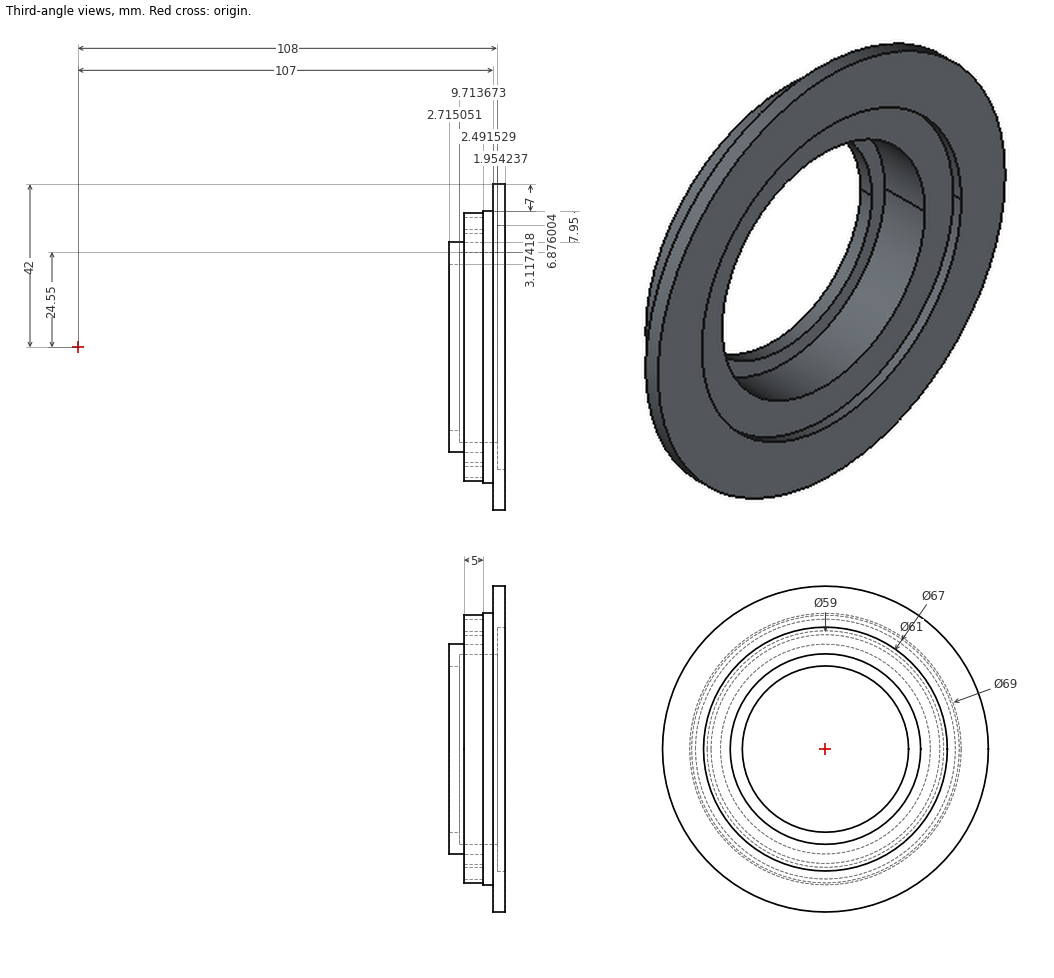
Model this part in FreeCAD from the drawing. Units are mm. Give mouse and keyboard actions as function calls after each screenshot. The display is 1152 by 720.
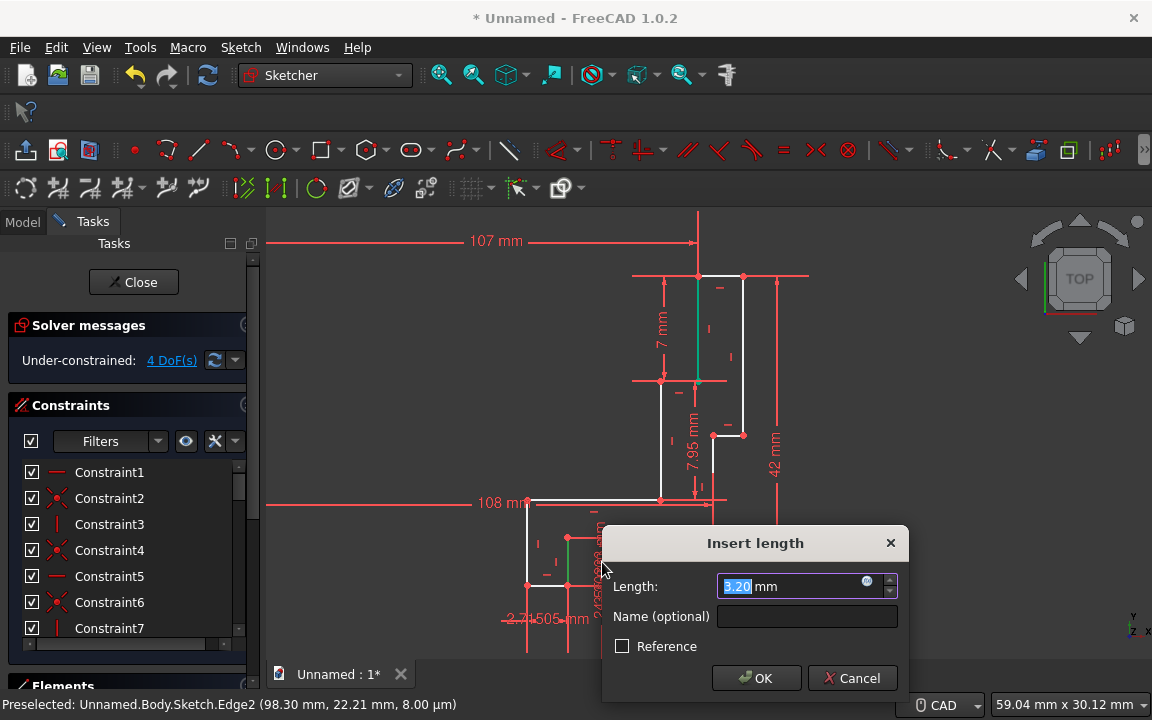
text(3.117418)
key(Return)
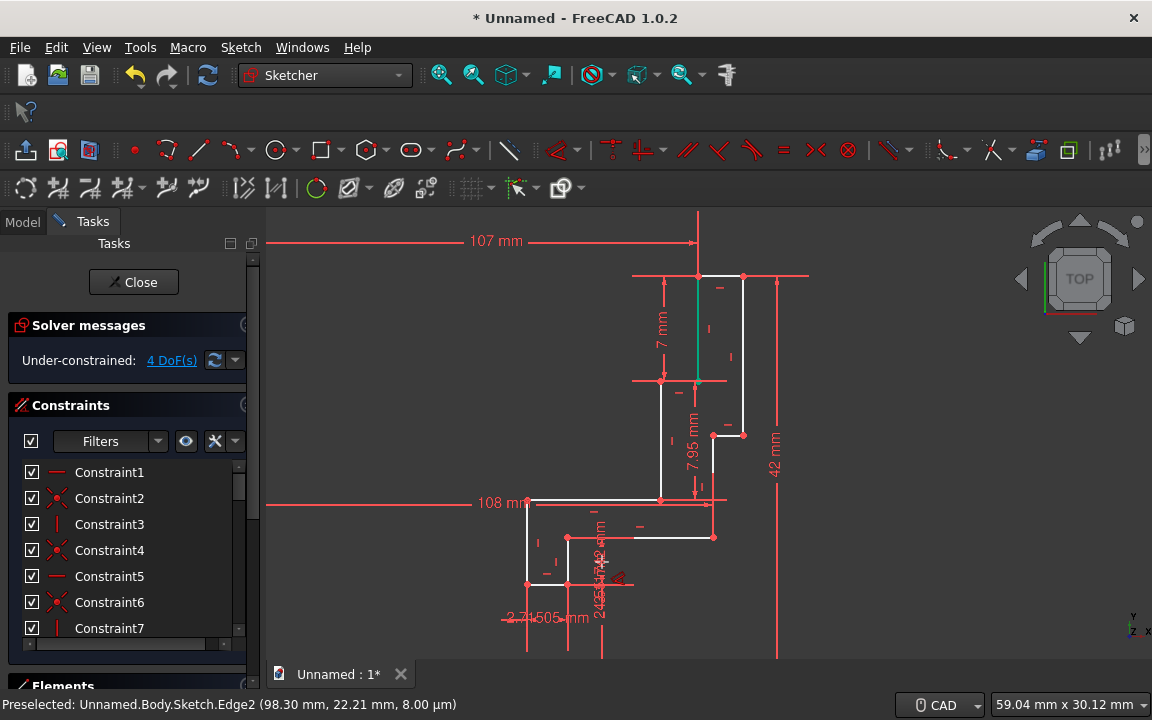
click(611, 538)
click(674, 572)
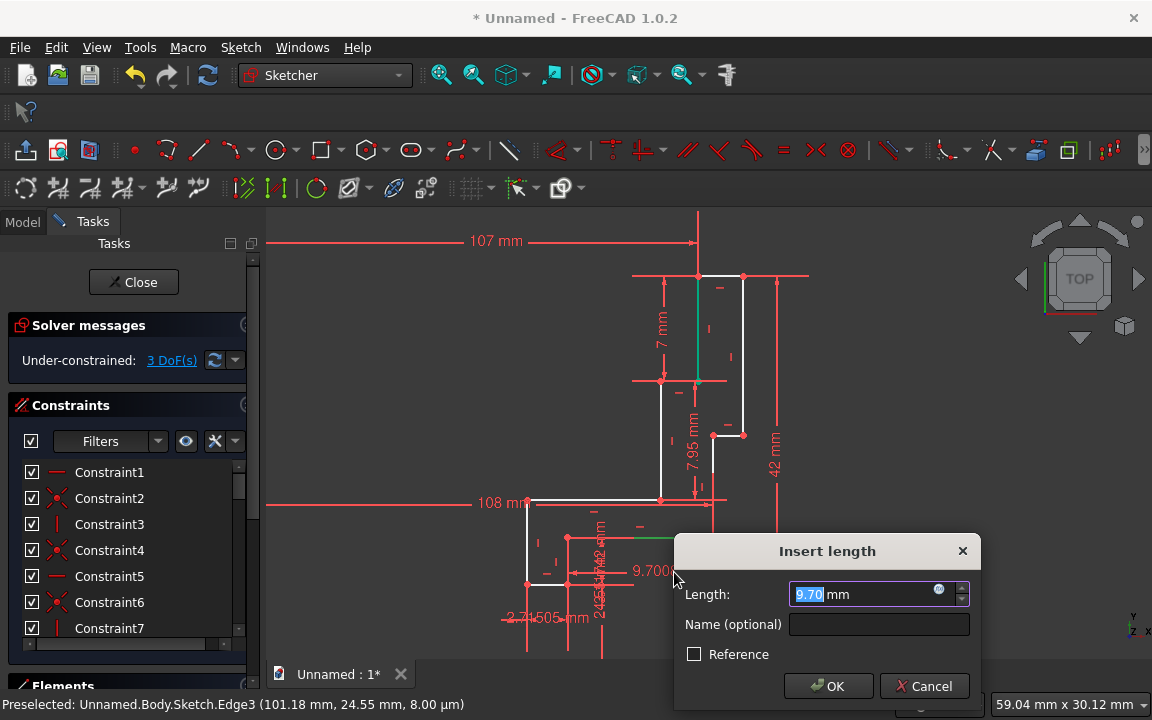
text(9.713673)
key(Return)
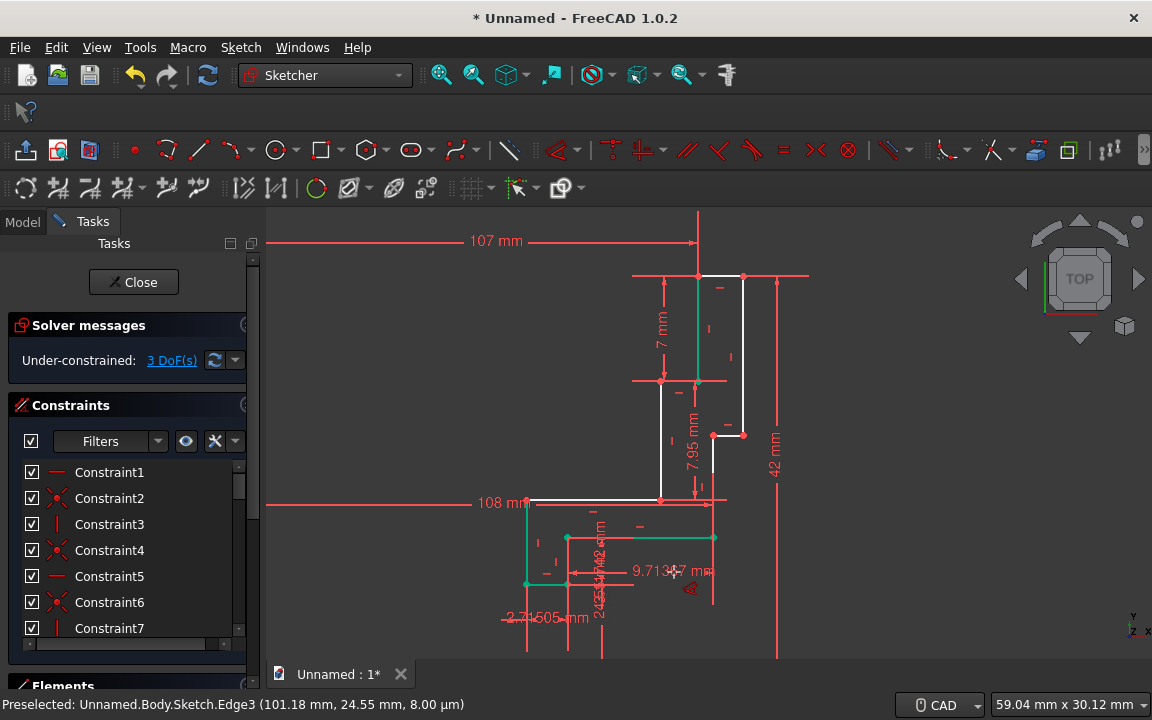
click(713, 507)
click(747, 487)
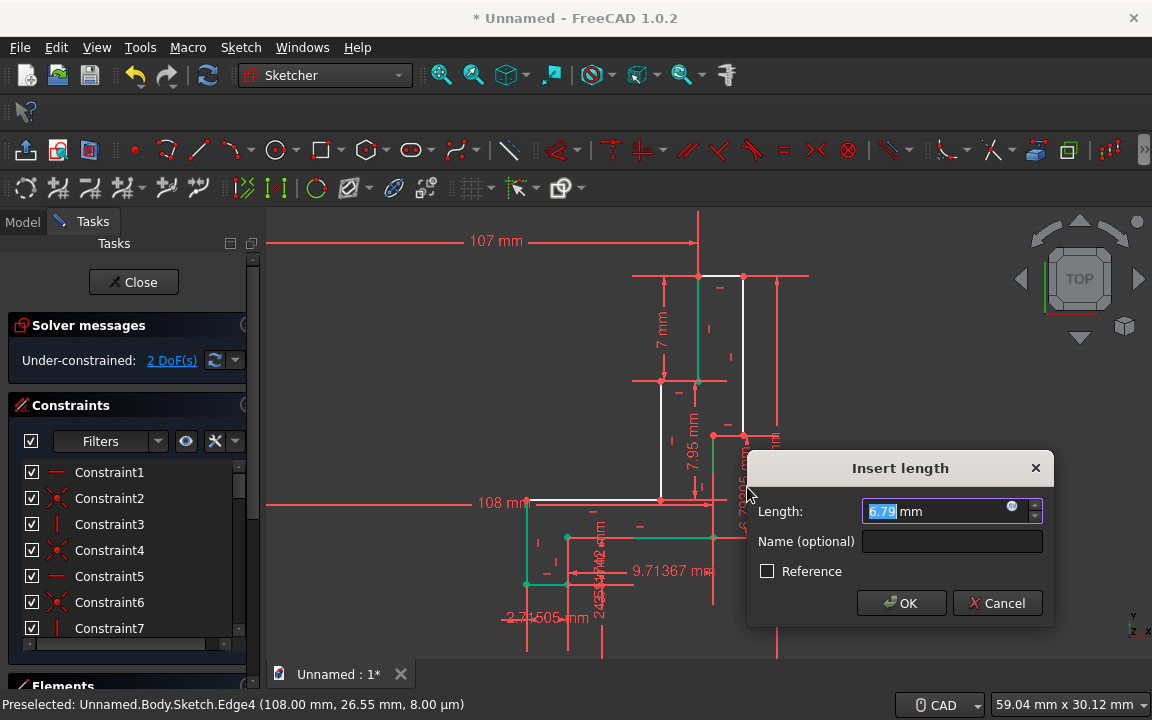
text(6.876004)
key(Return)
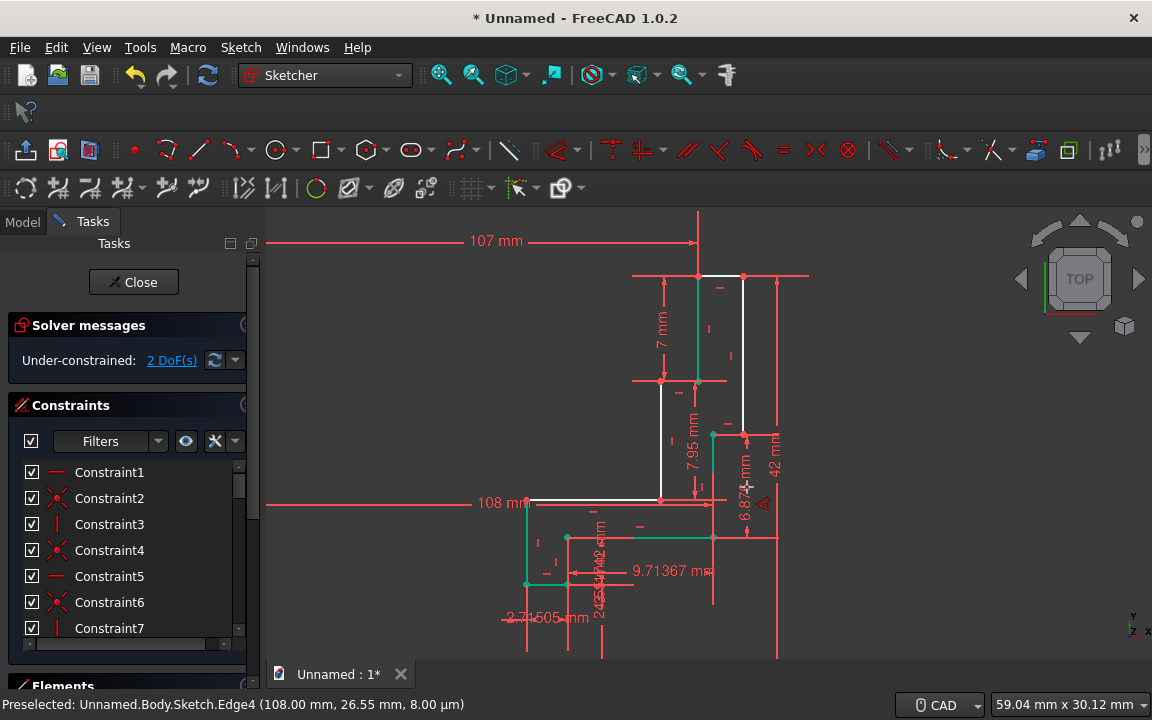
scroll(725, 435, up, 2)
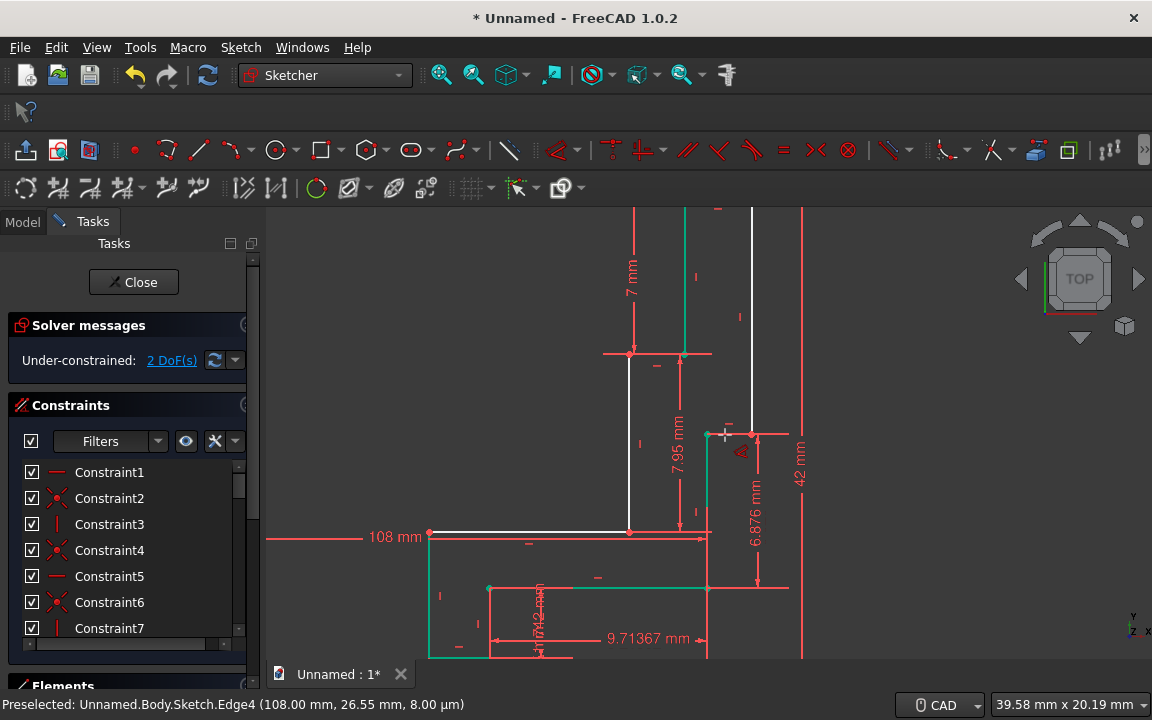
click(725, 434)
click(729, 468)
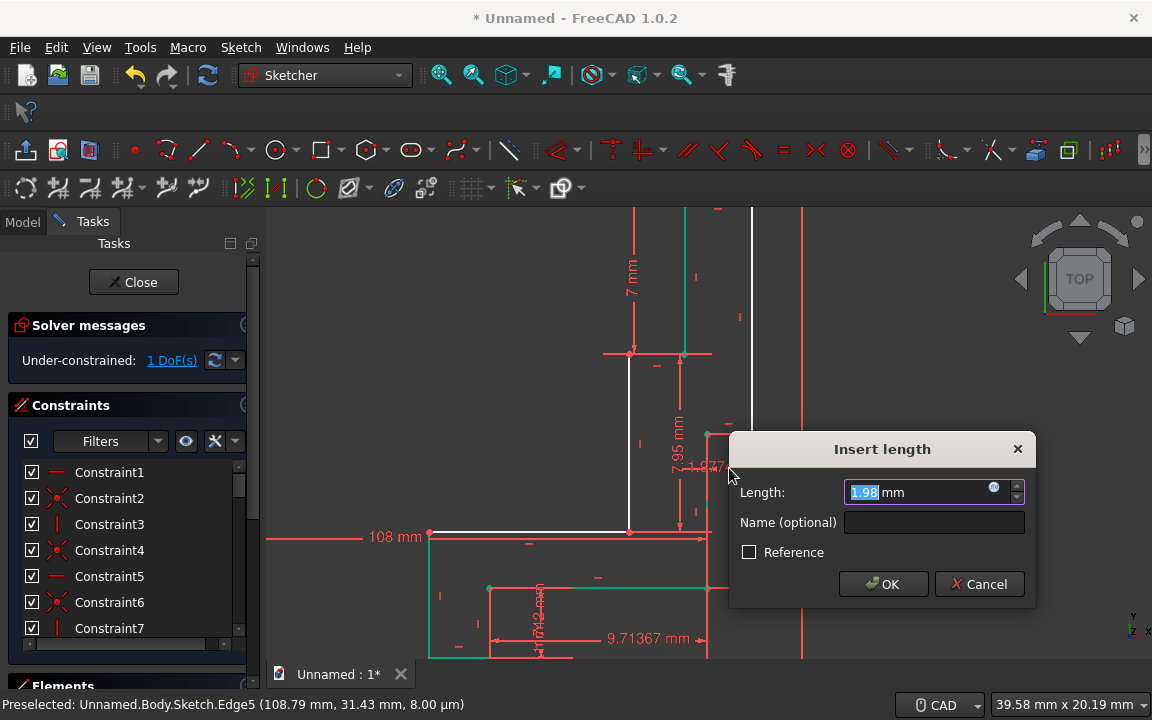
text(1.954237)
key(Return)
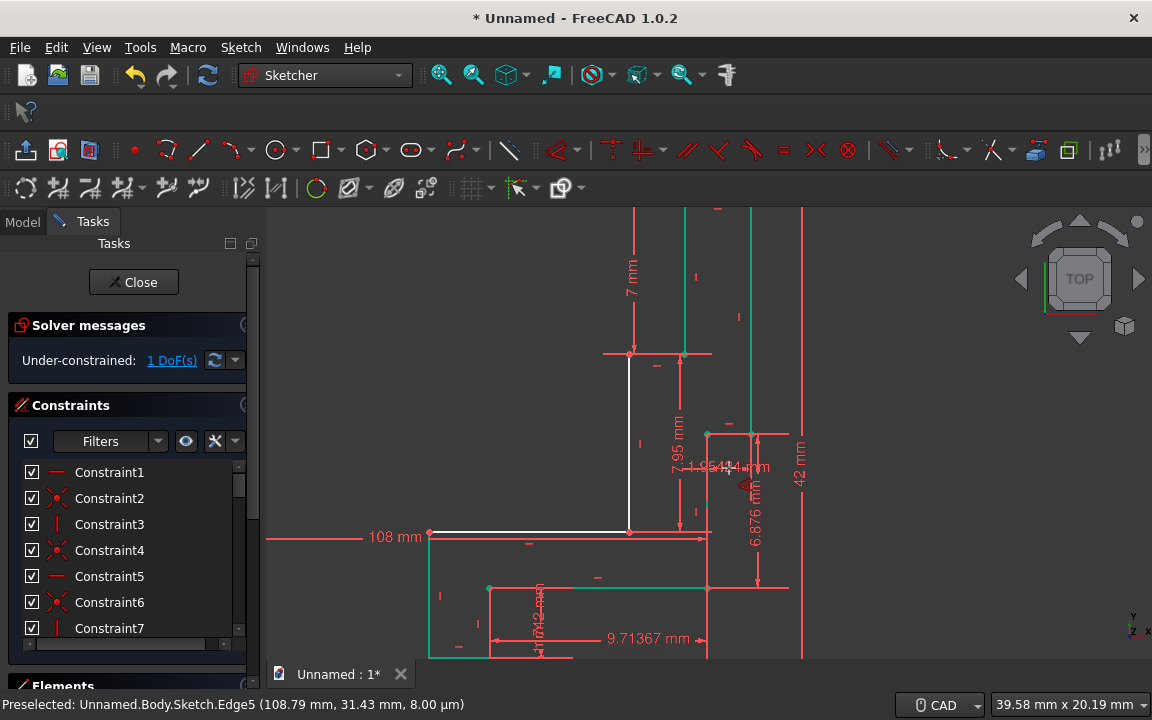
click(668, 354)
click(657, 320)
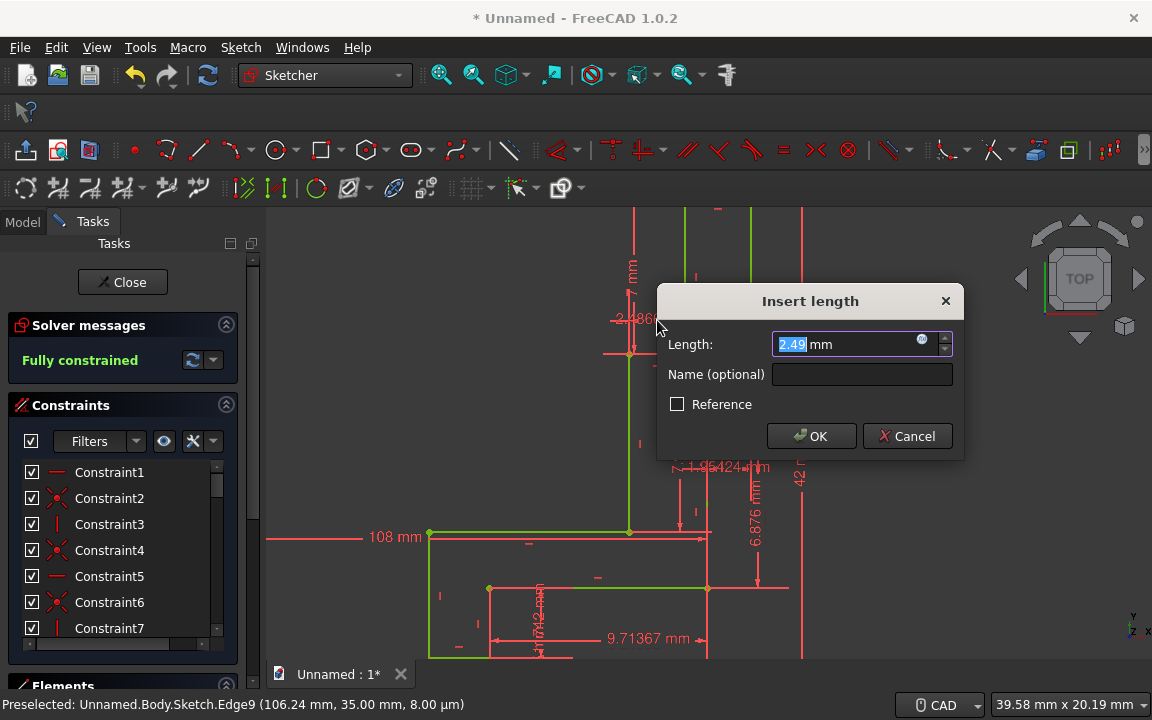
text(2.491529)
key(Return)
key(Escape)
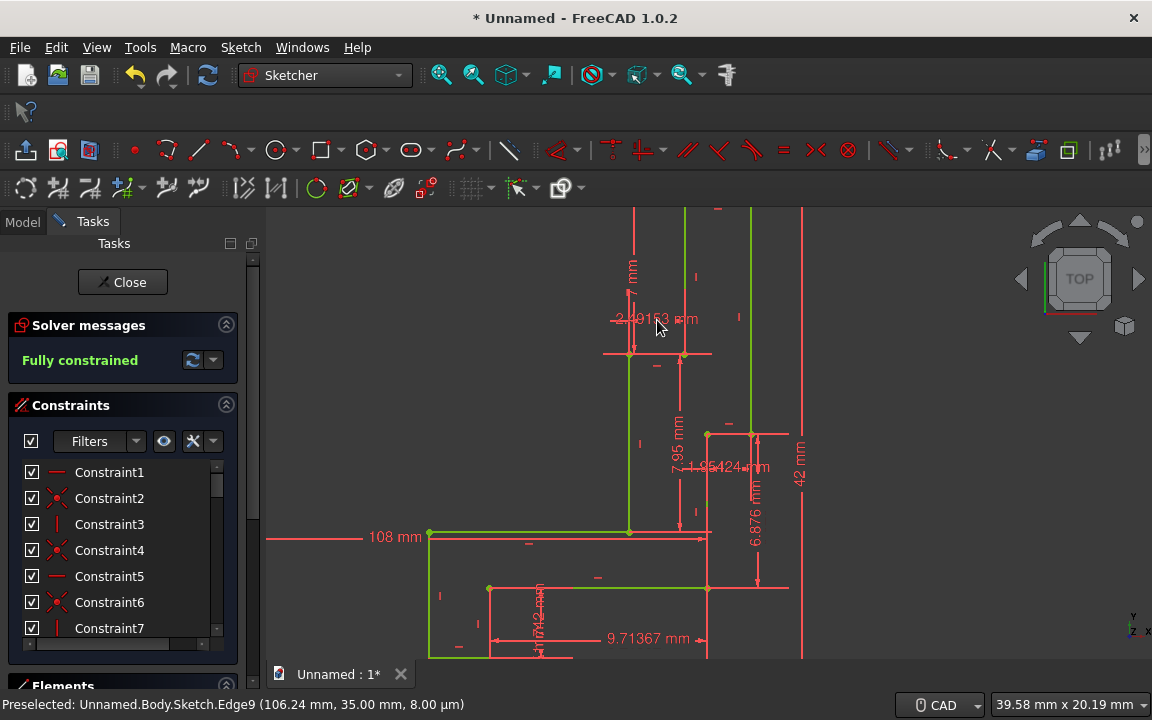
click(123, 282)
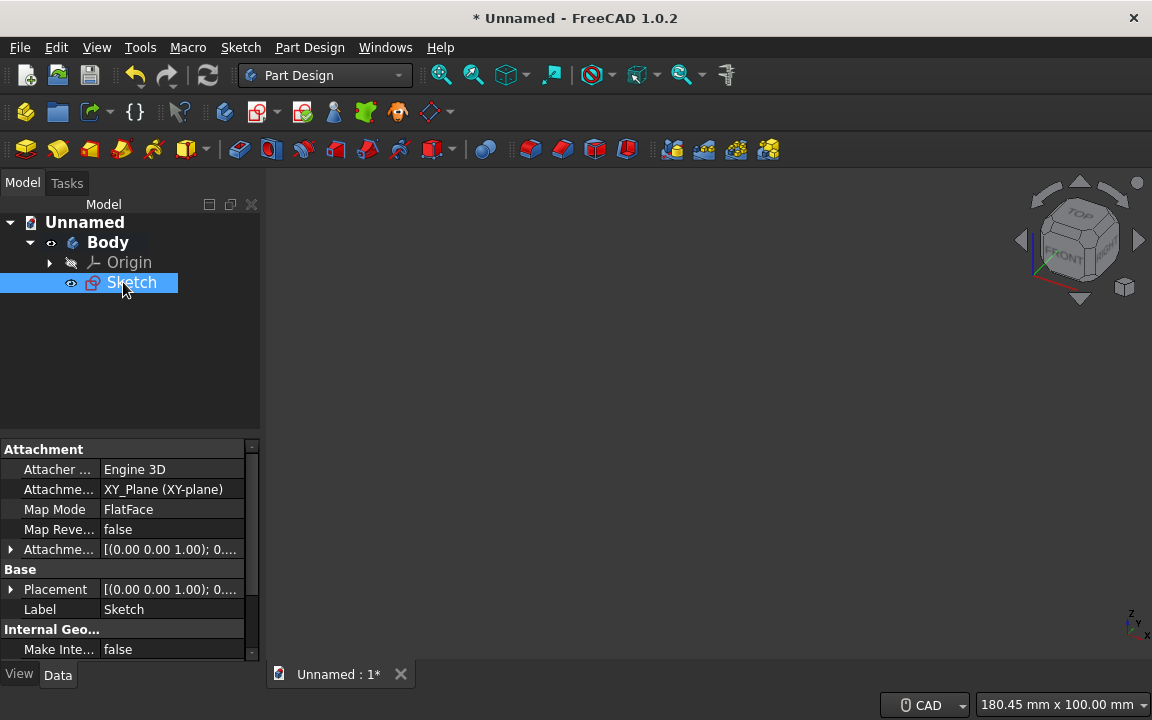
click(58, 150)